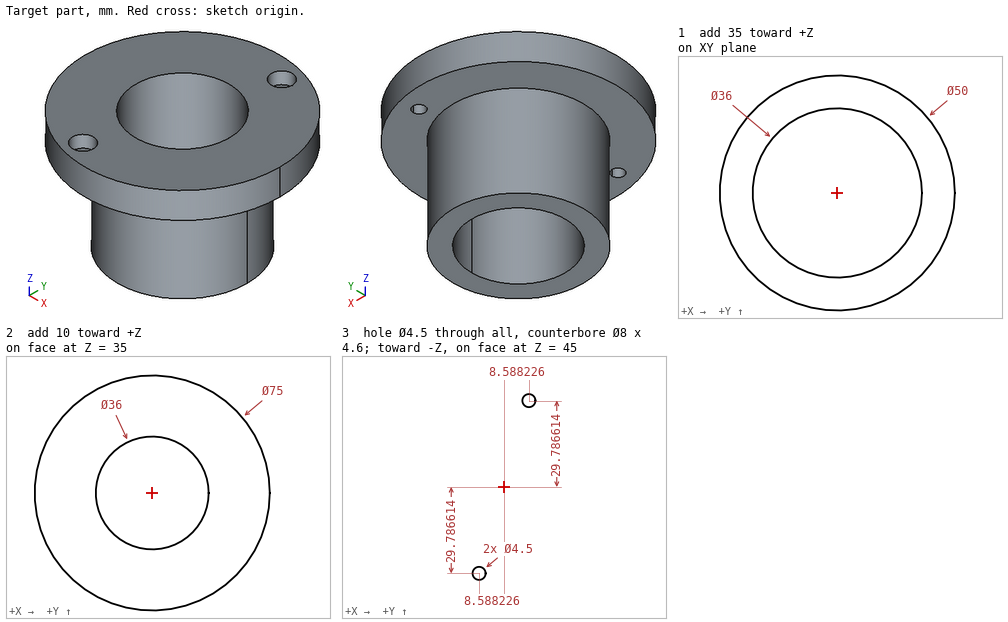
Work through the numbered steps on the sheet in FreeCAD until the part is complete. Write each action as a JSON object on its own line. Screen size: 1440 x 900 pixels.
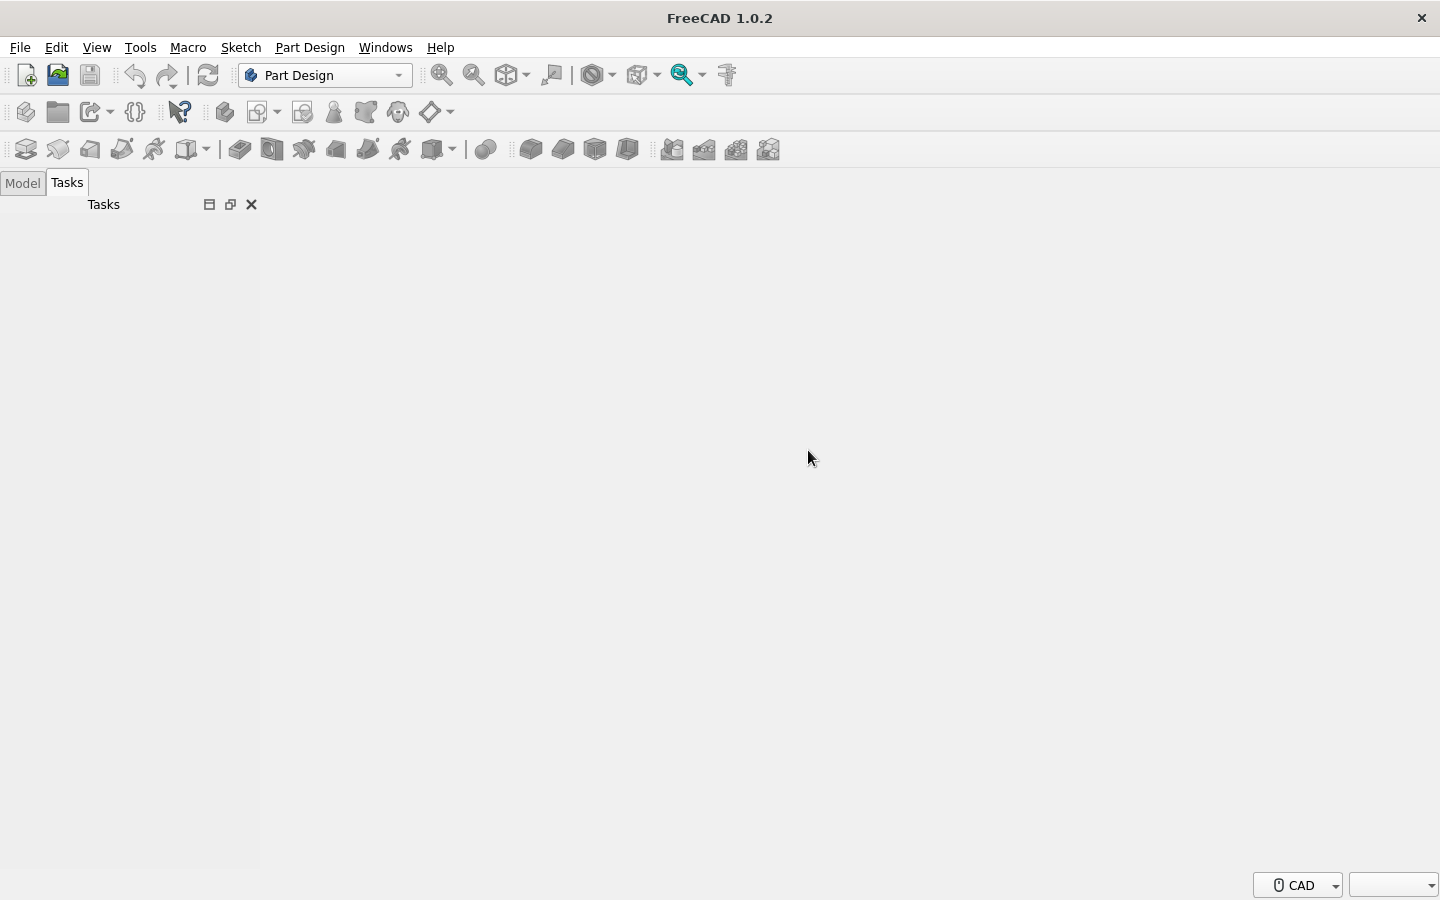
{"action": "left_click", "coordinate": [26, 76]}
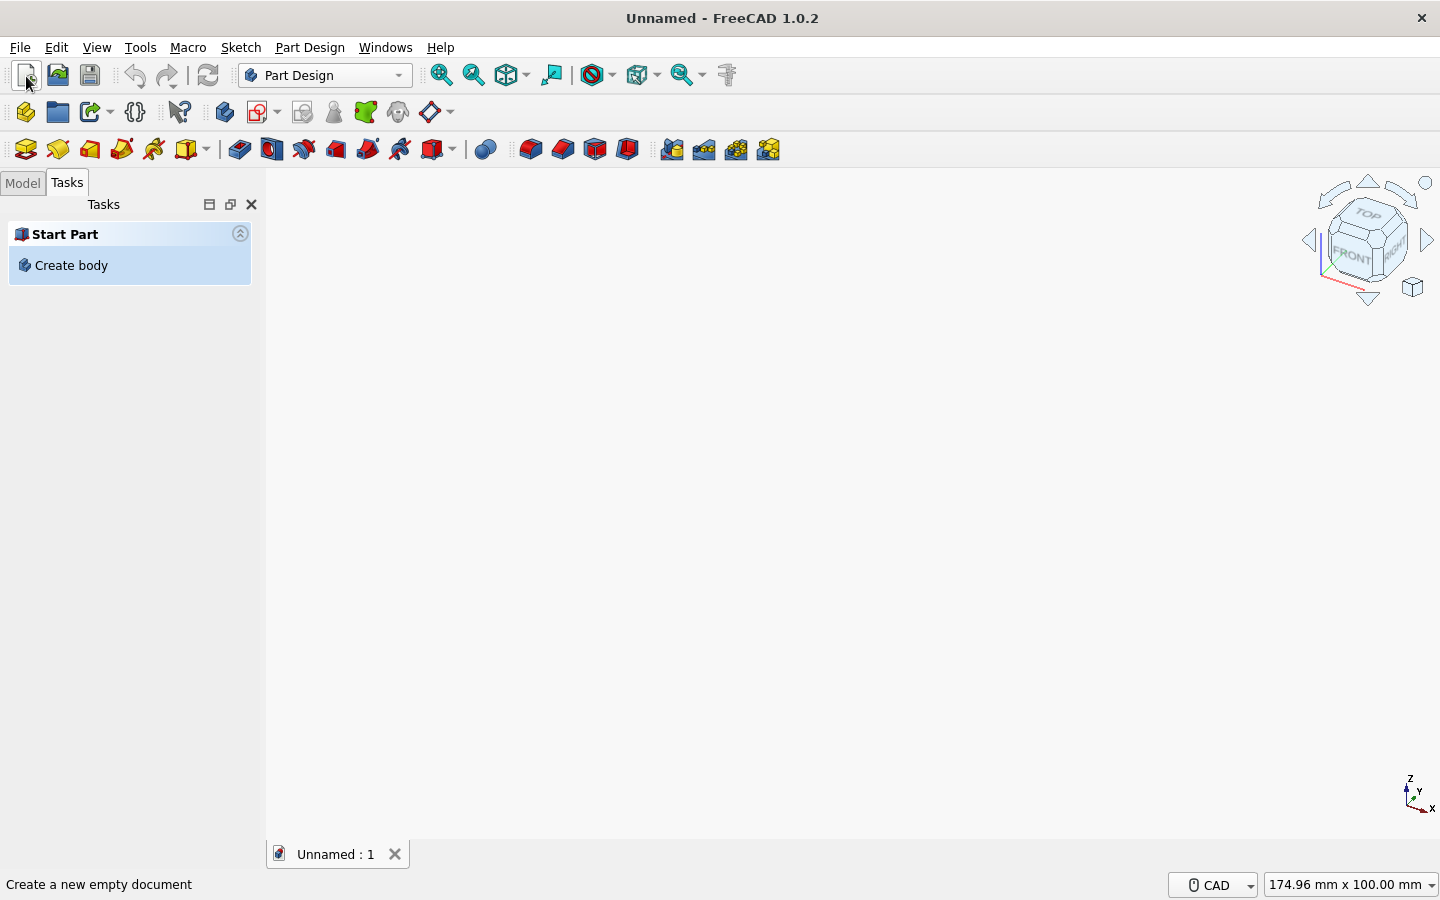
{"action": "left_click", "coordinate": [258, 112]}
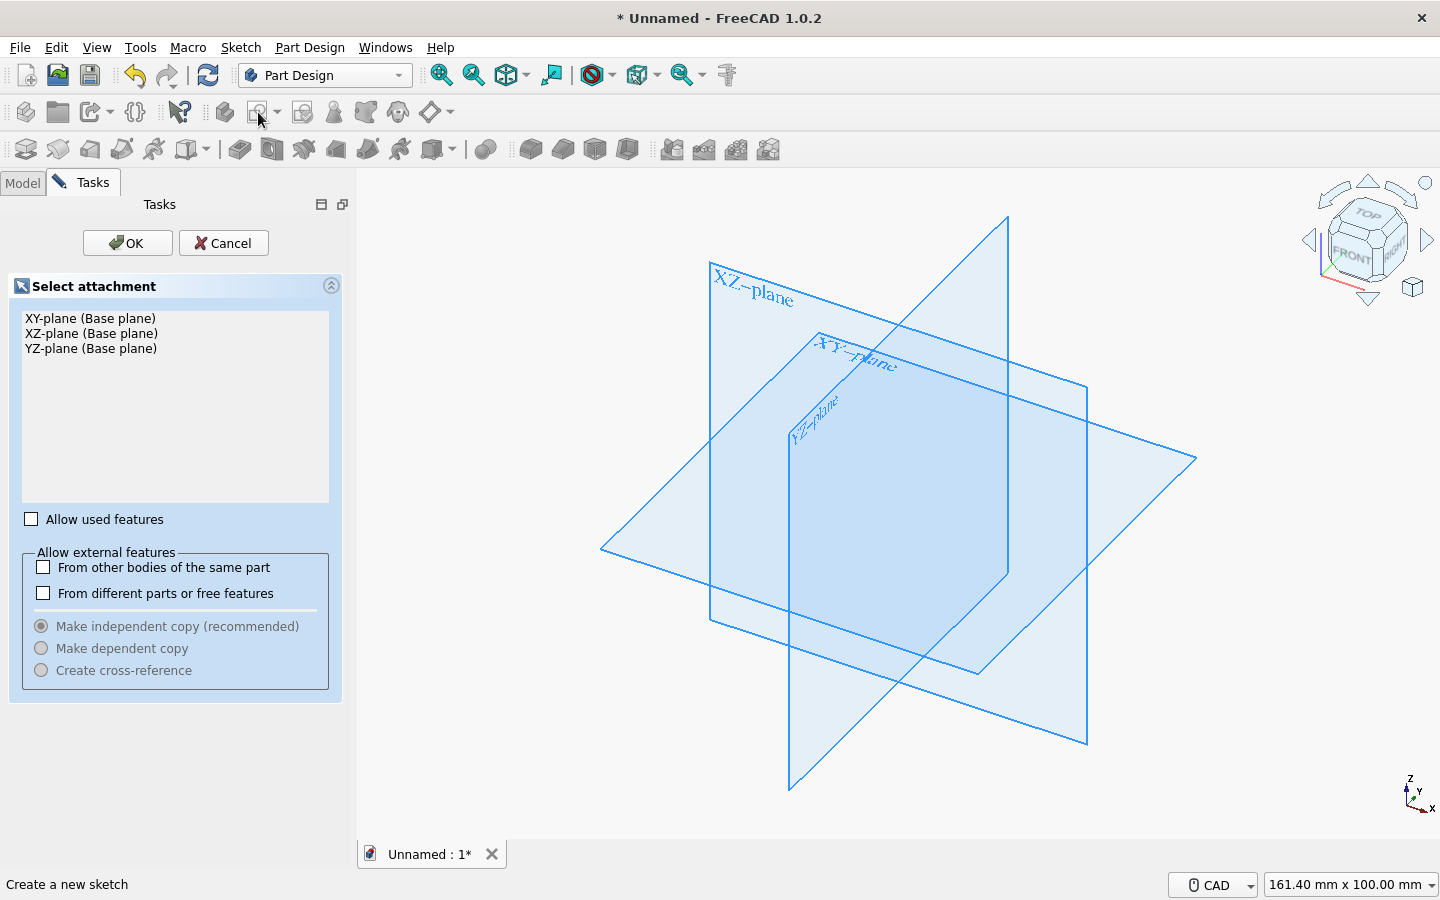
{"action": "left_click", "coordinate": [82, 318]}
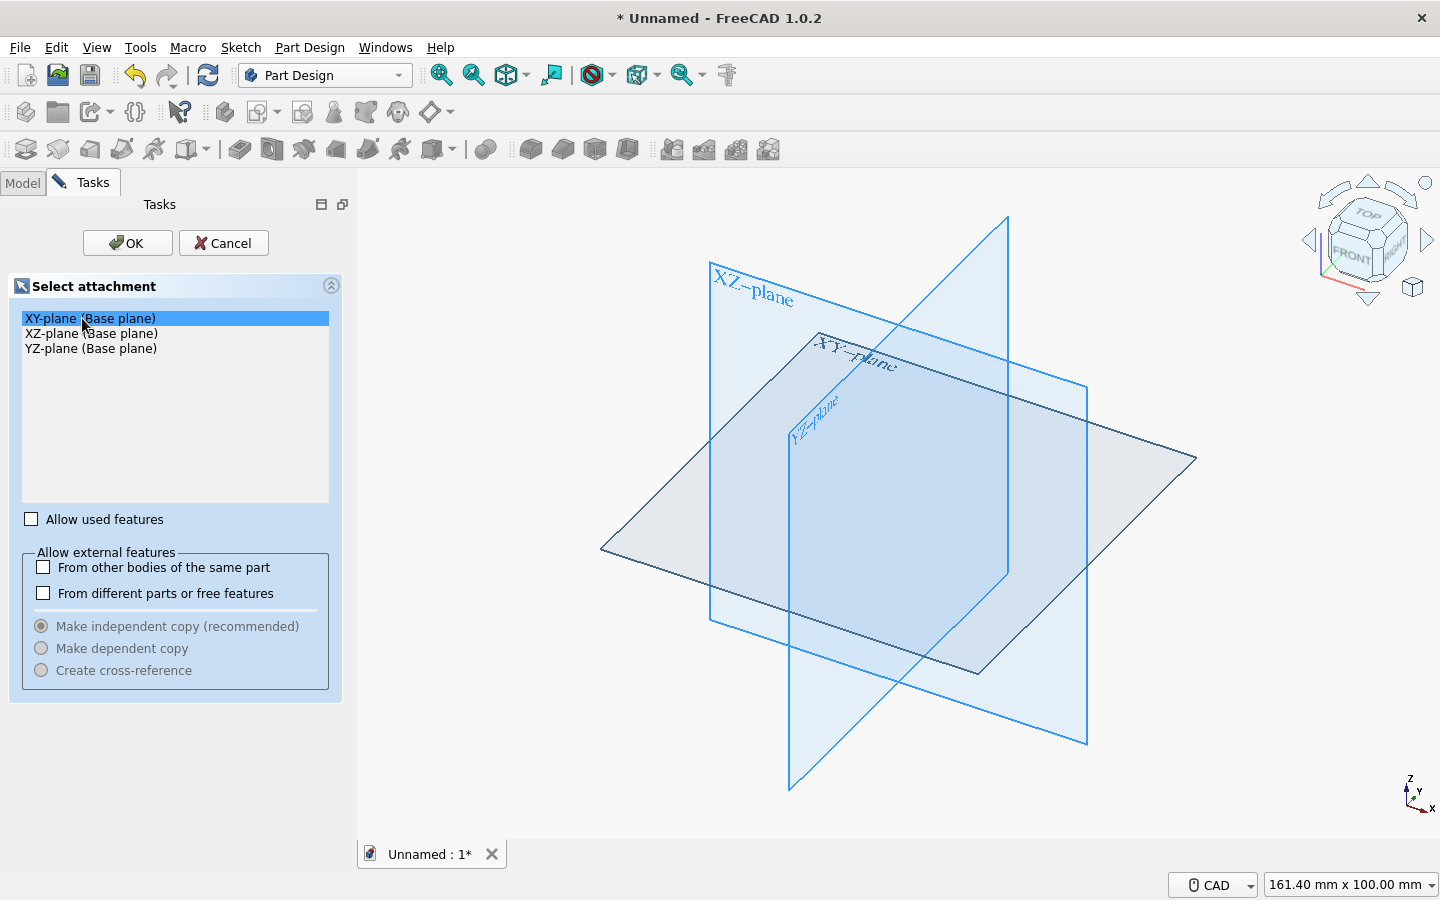
{"action": "left_click", "coordinate": [128, 243]}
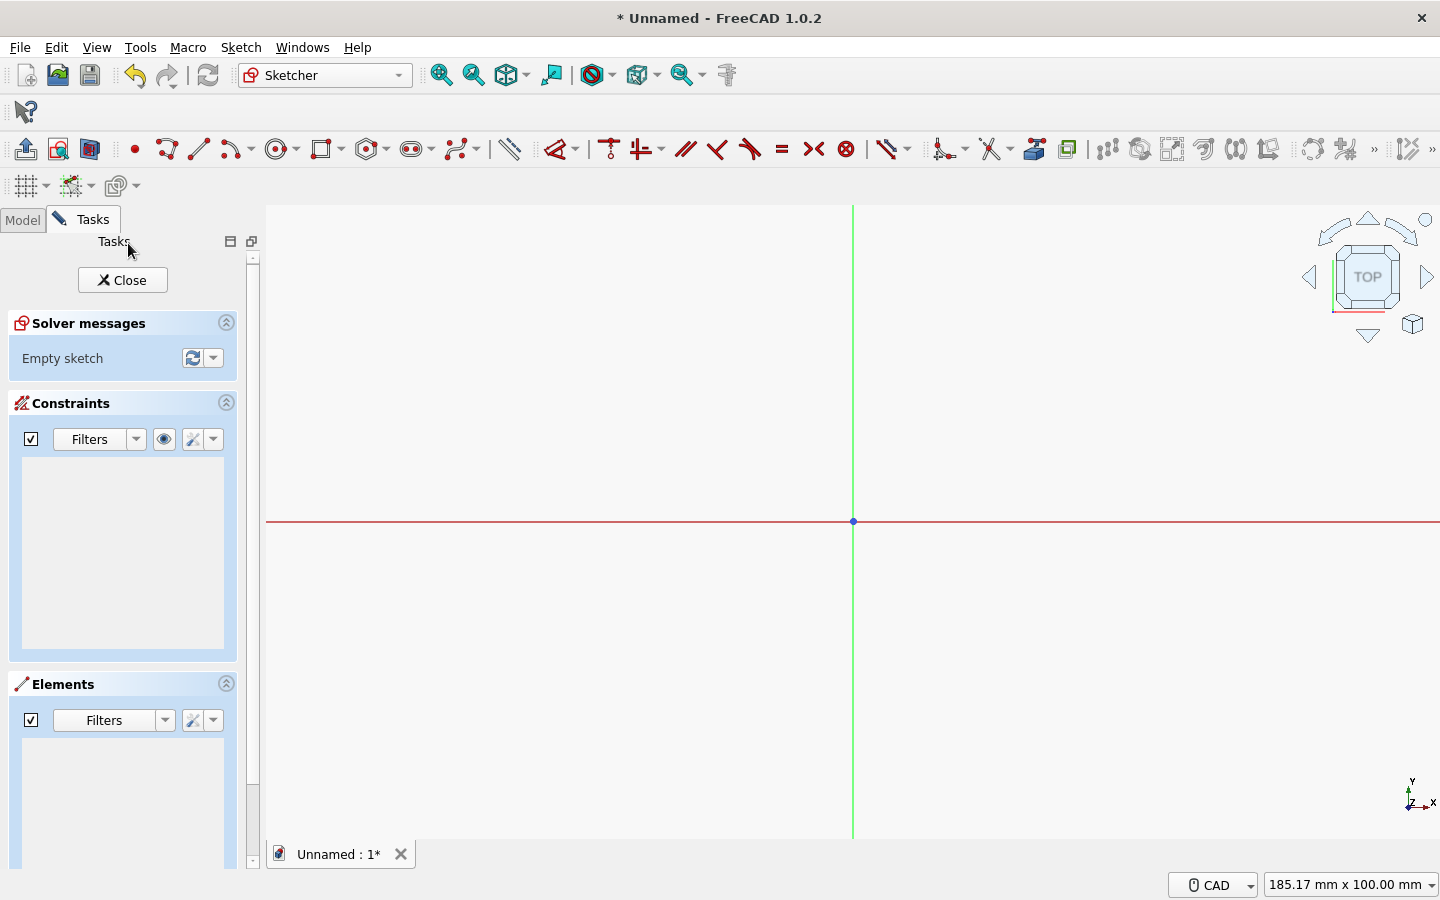
{"action": "left_click", "coordinate": [276, 150]}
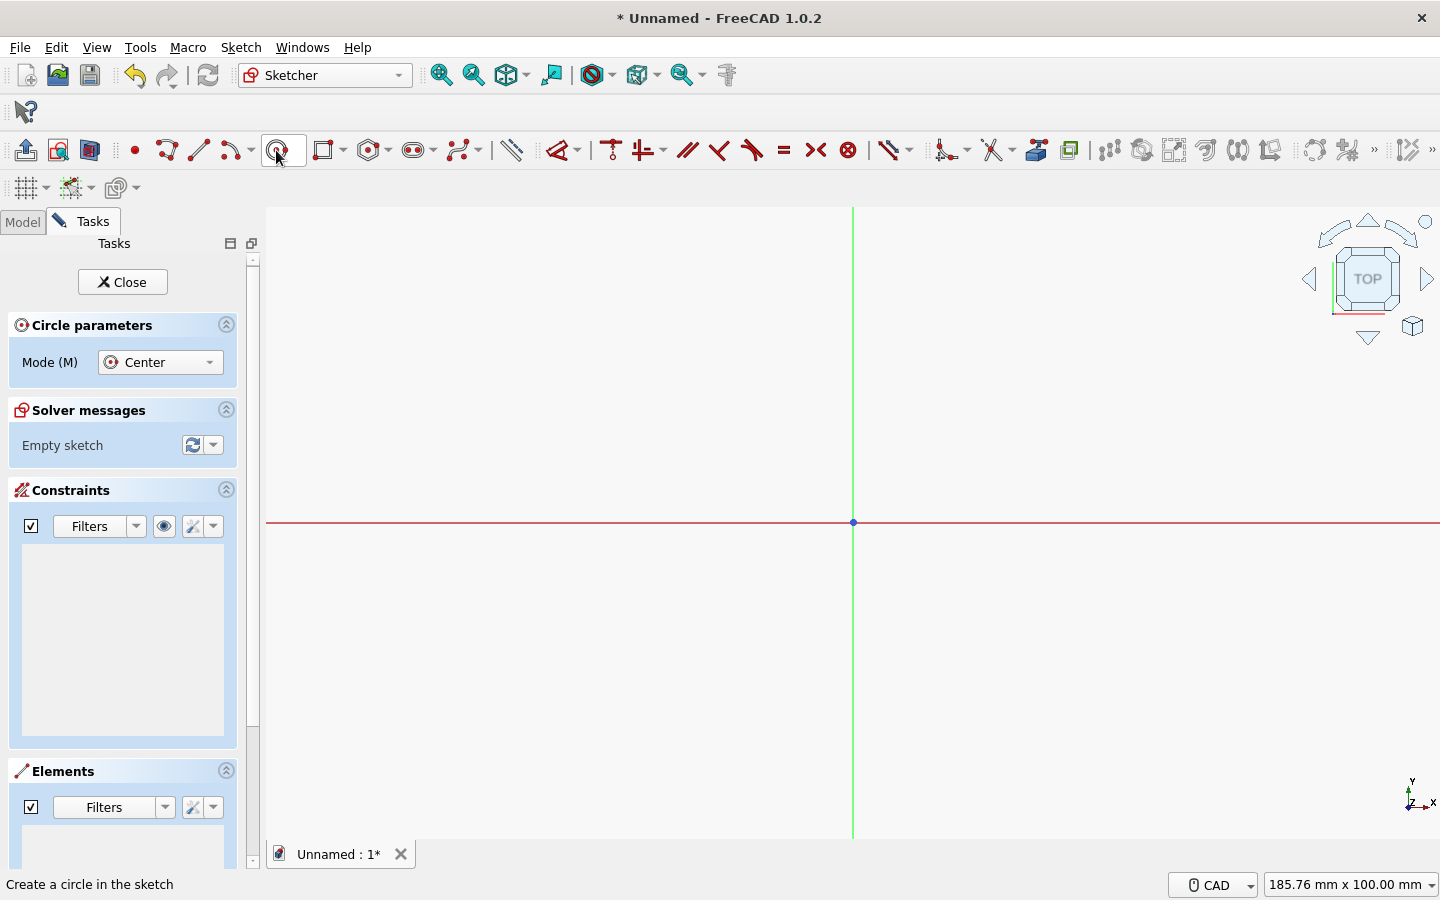
{"action": "left_click", "coordinate": [853, 523]}
{"action": "left_click", "coordinate": [965, 411]}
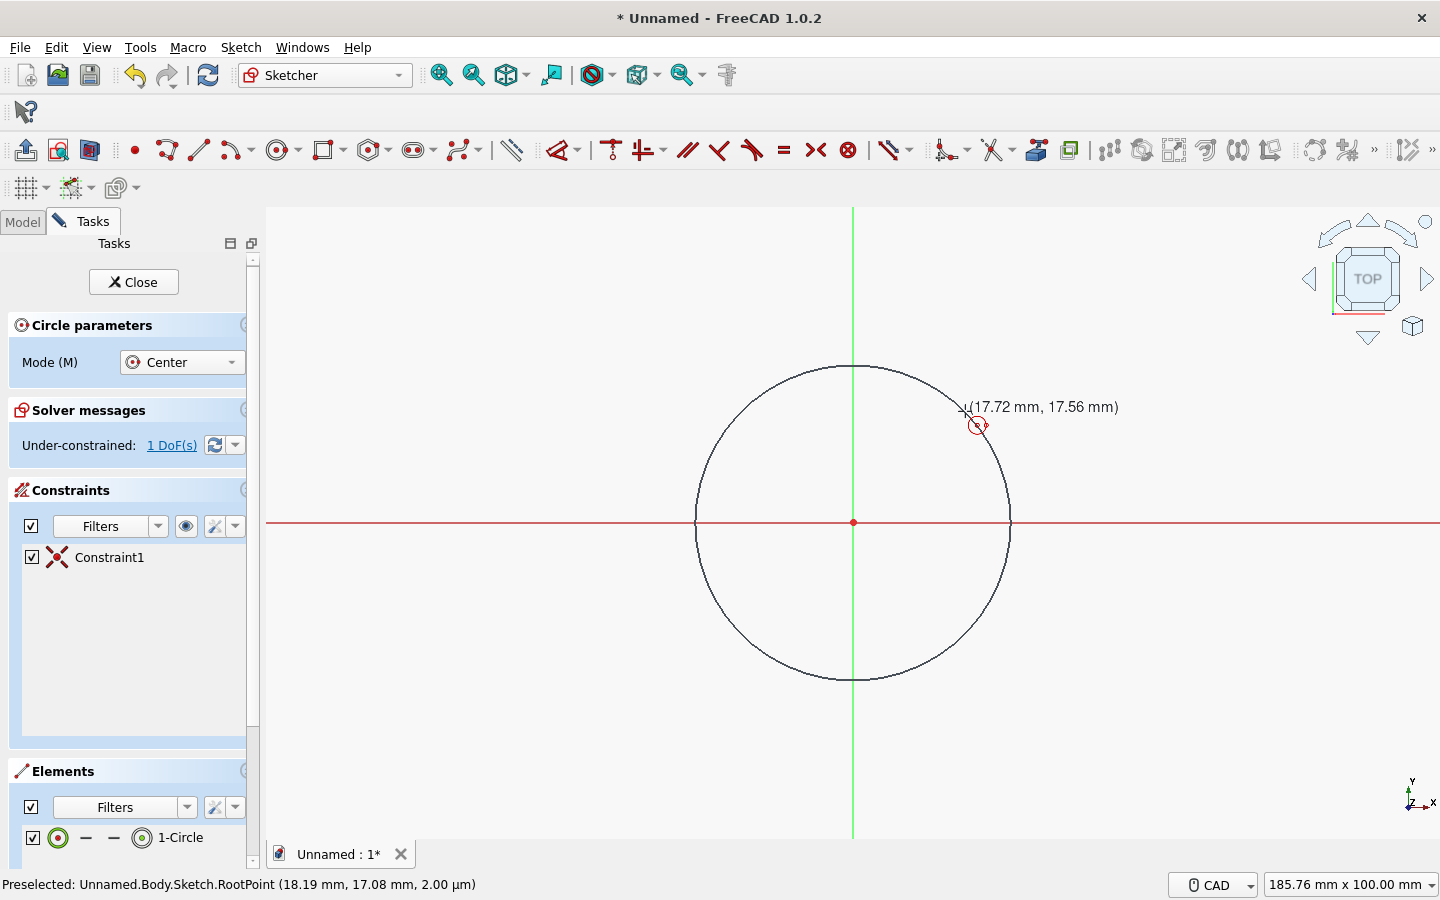
{"action": "left_click", "coordinate": [853, 523]}
{"action": "left_click", "coordinate": [933, 443]}
{"action": "key", "text": "Escape"}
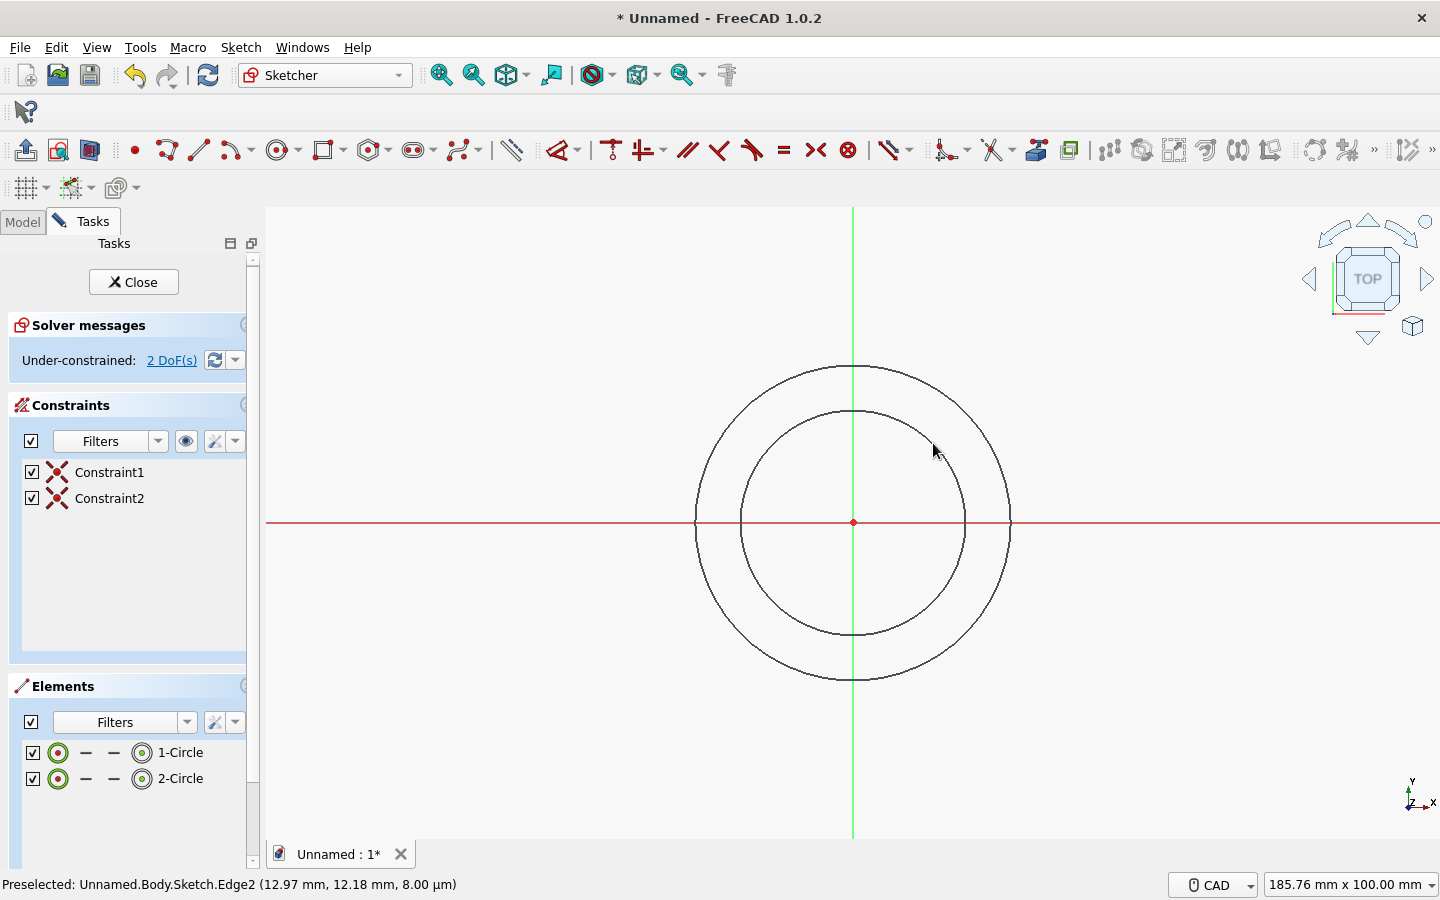
{"action": "left_click", "coordinate": [558, 150]}